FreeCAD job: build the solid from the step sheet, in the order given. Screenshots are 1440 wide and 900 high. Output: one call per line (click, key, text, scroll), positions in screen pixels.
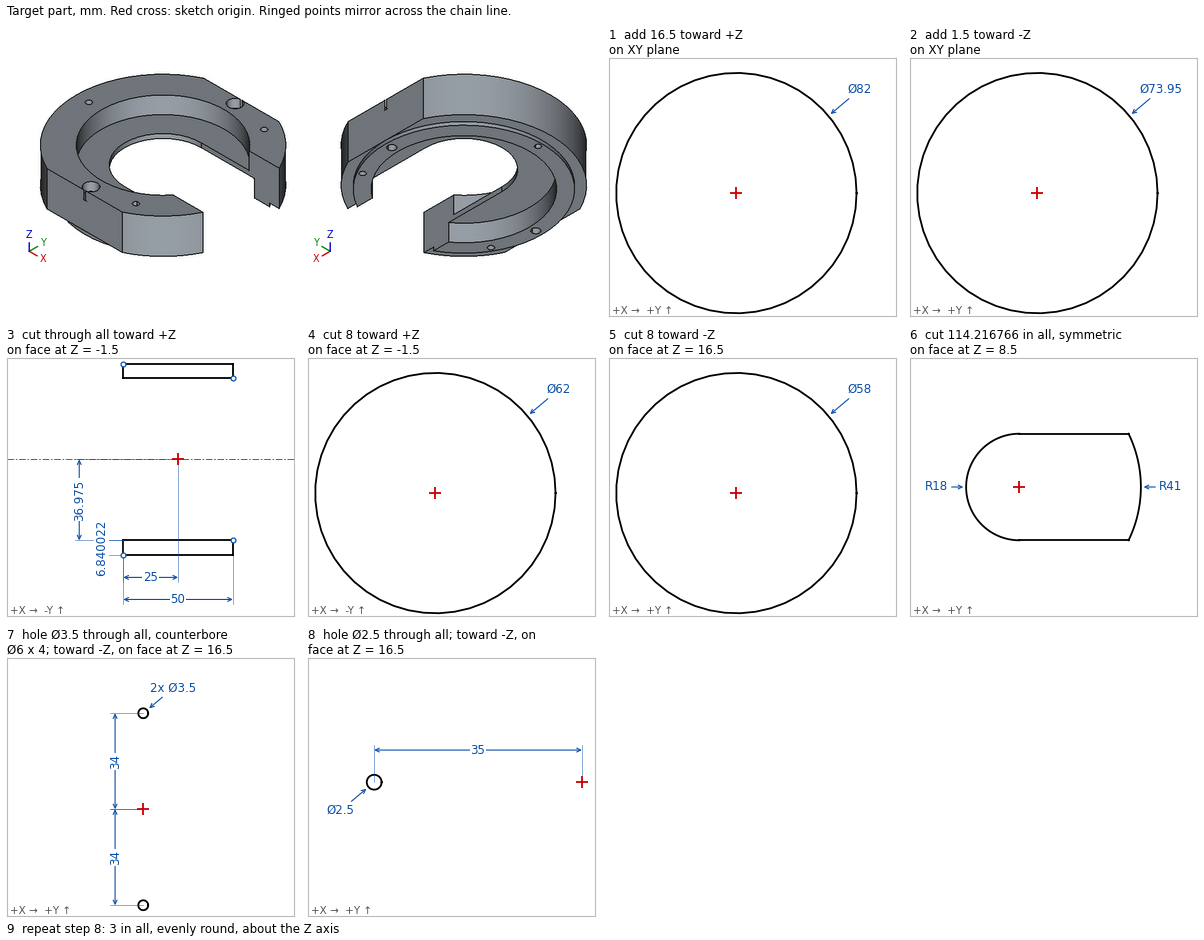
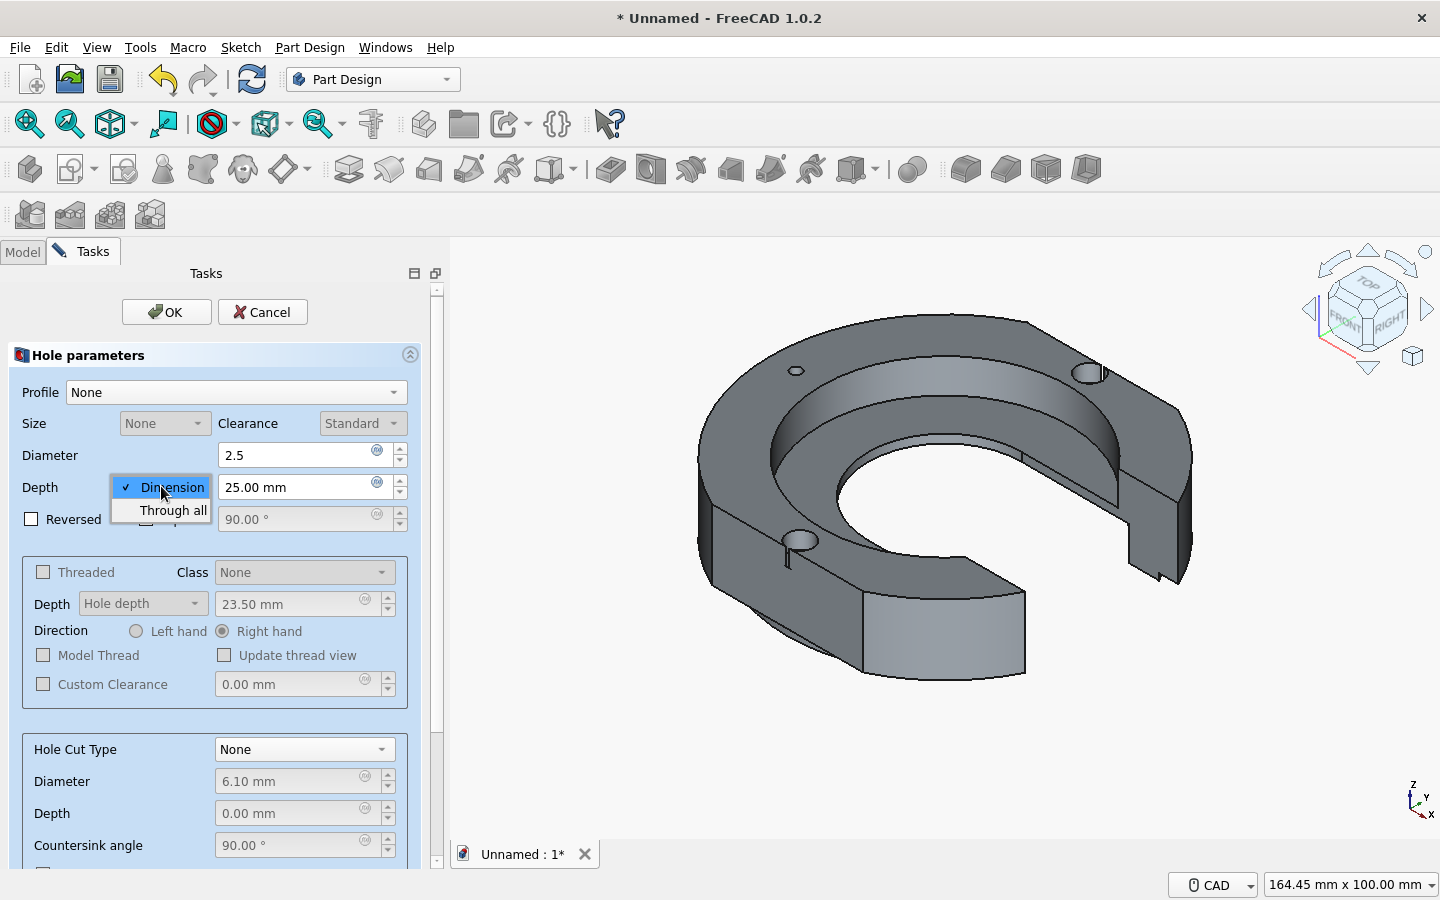
click(160, 510)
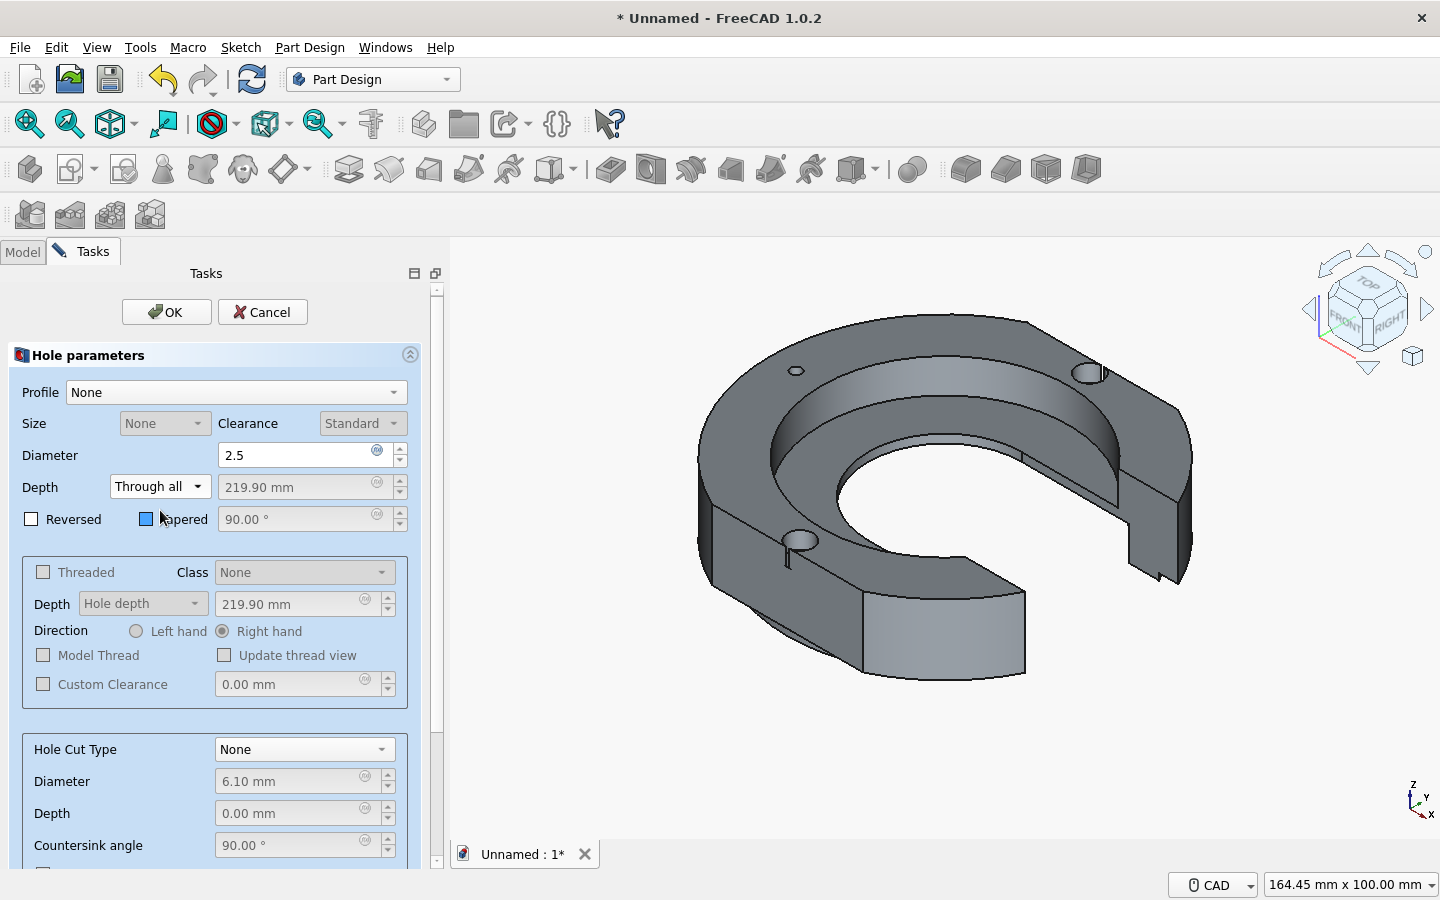
click(167, 312)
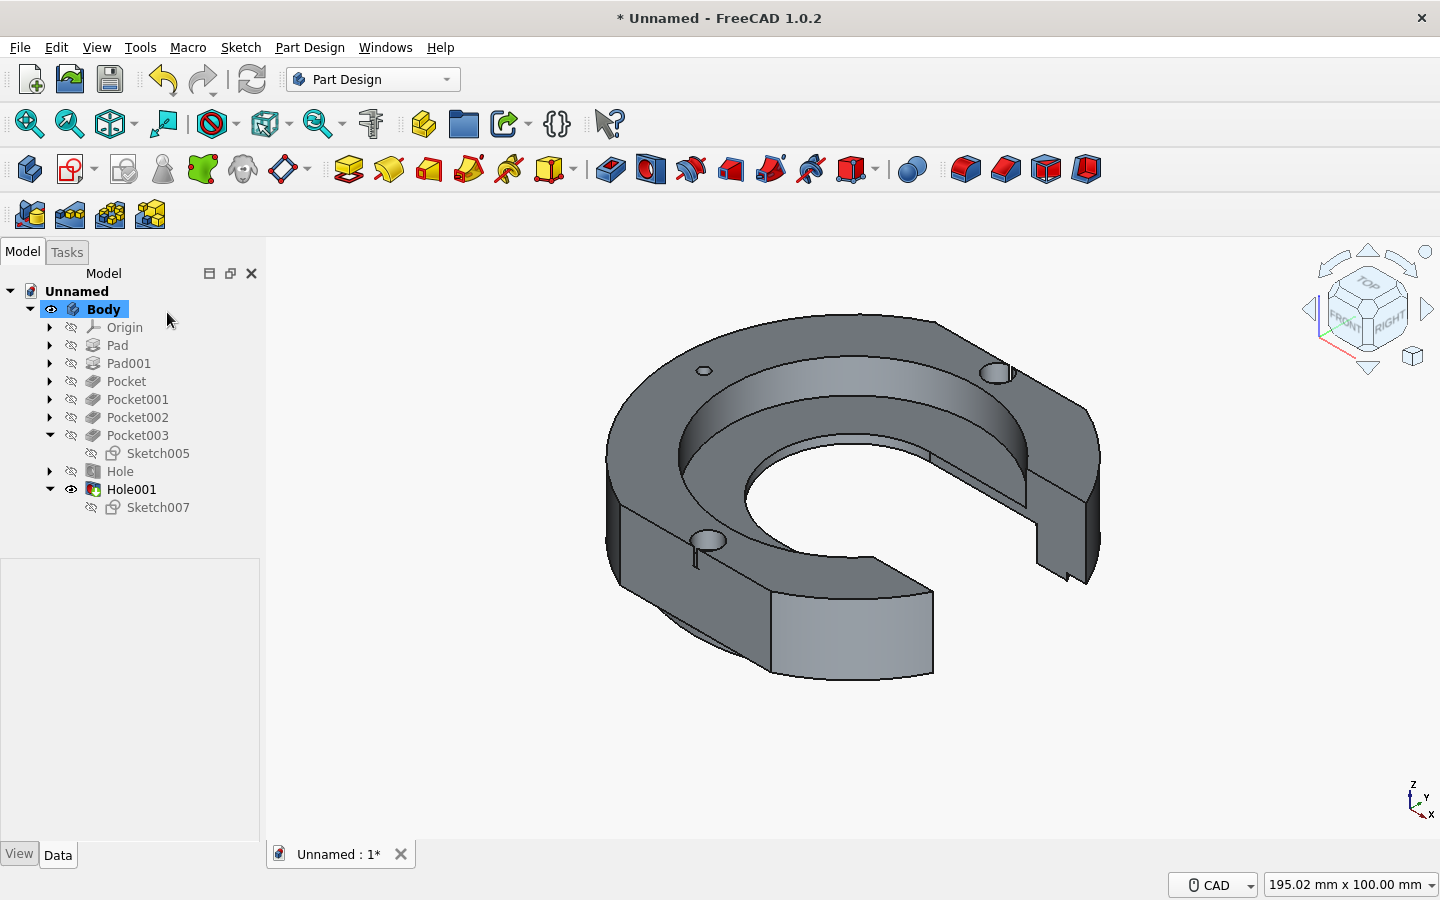
click(116, 489)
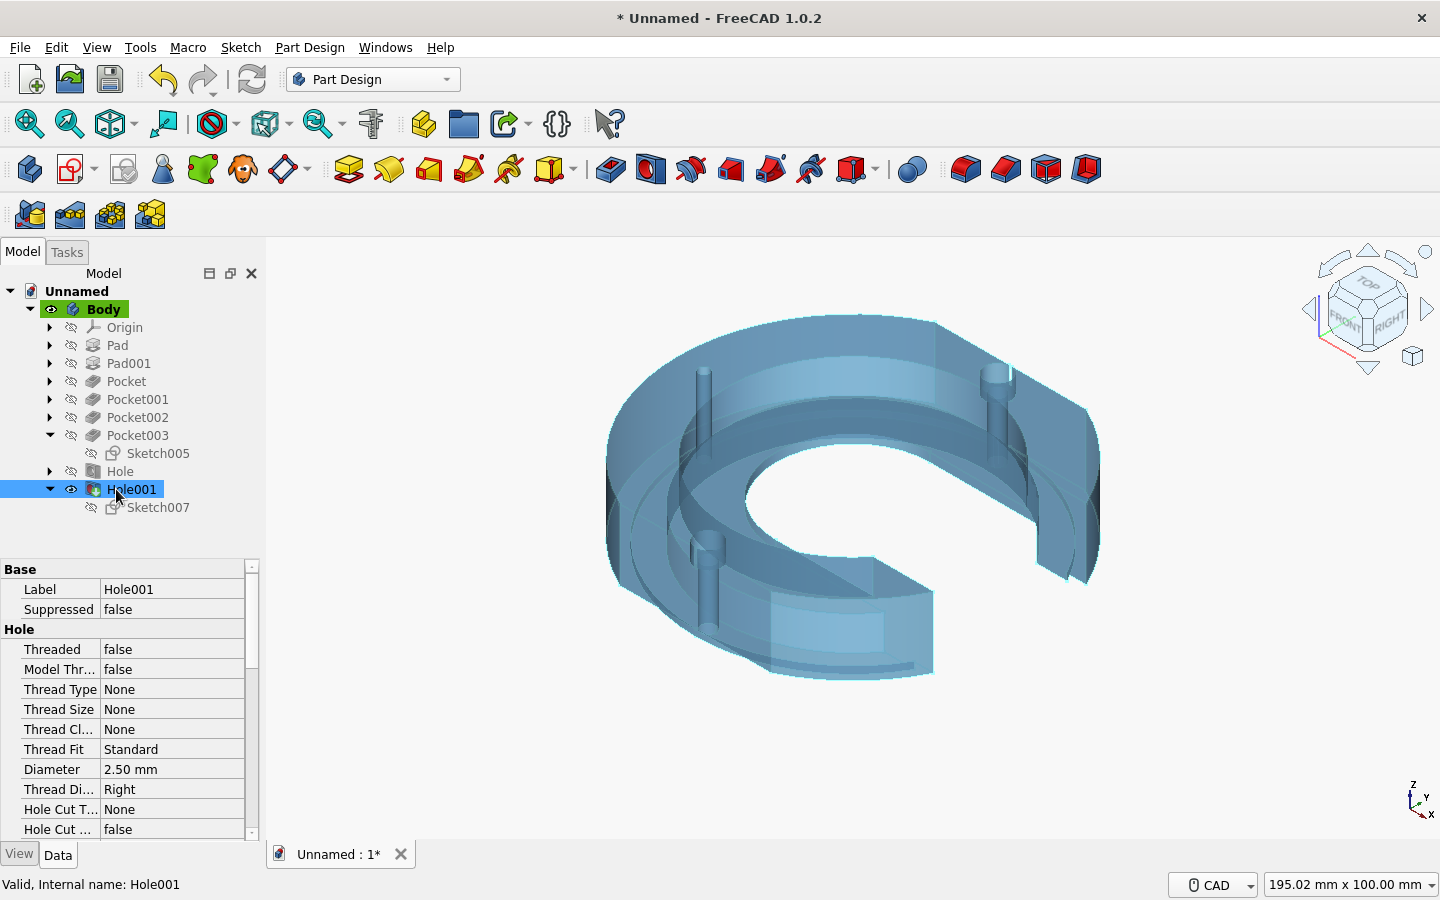
click(110, 214)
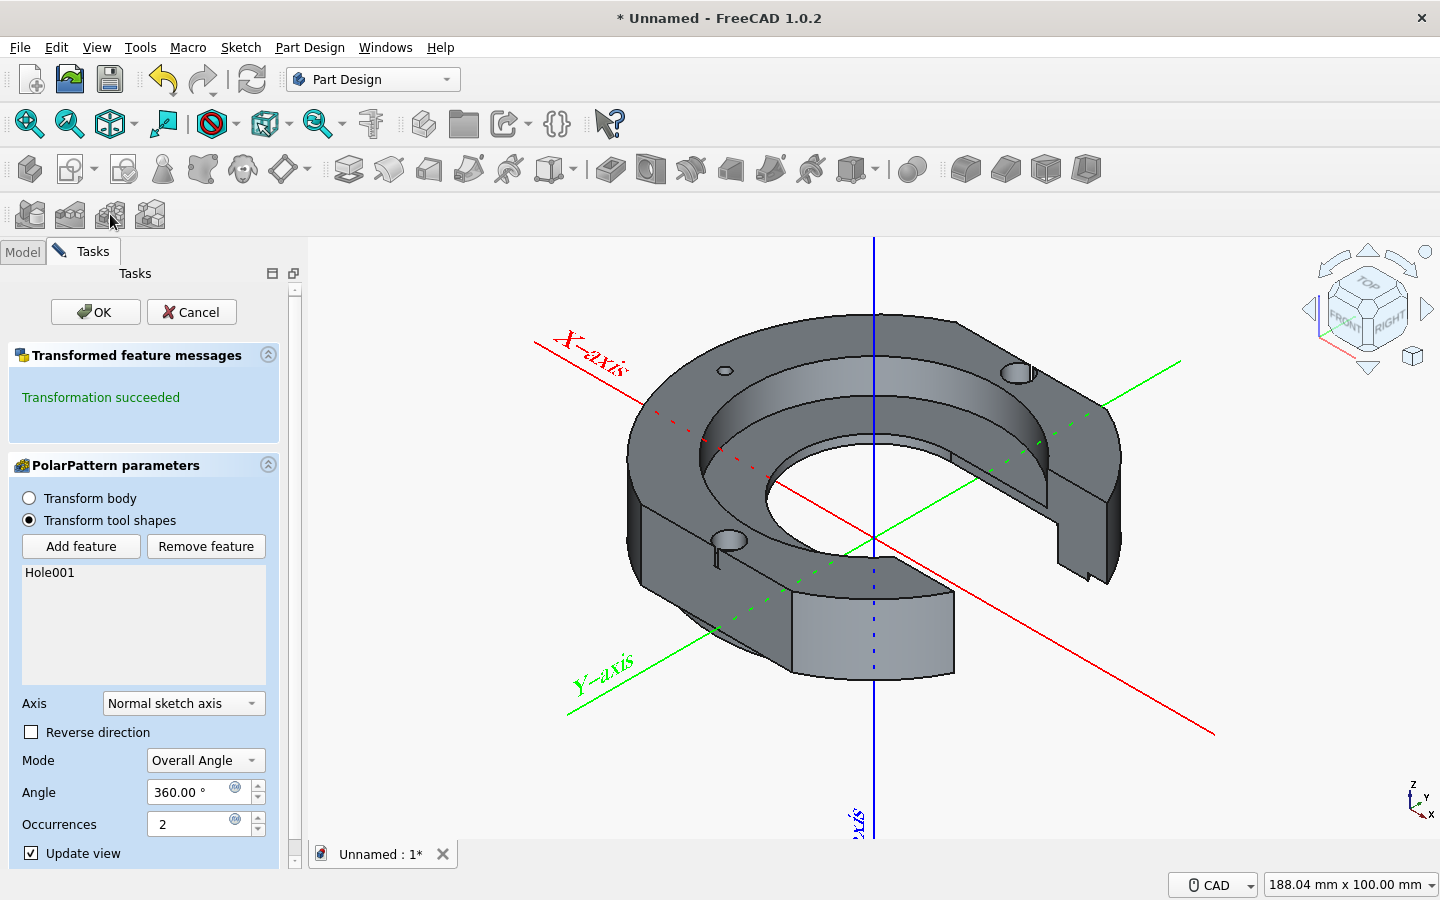
click(184, 704)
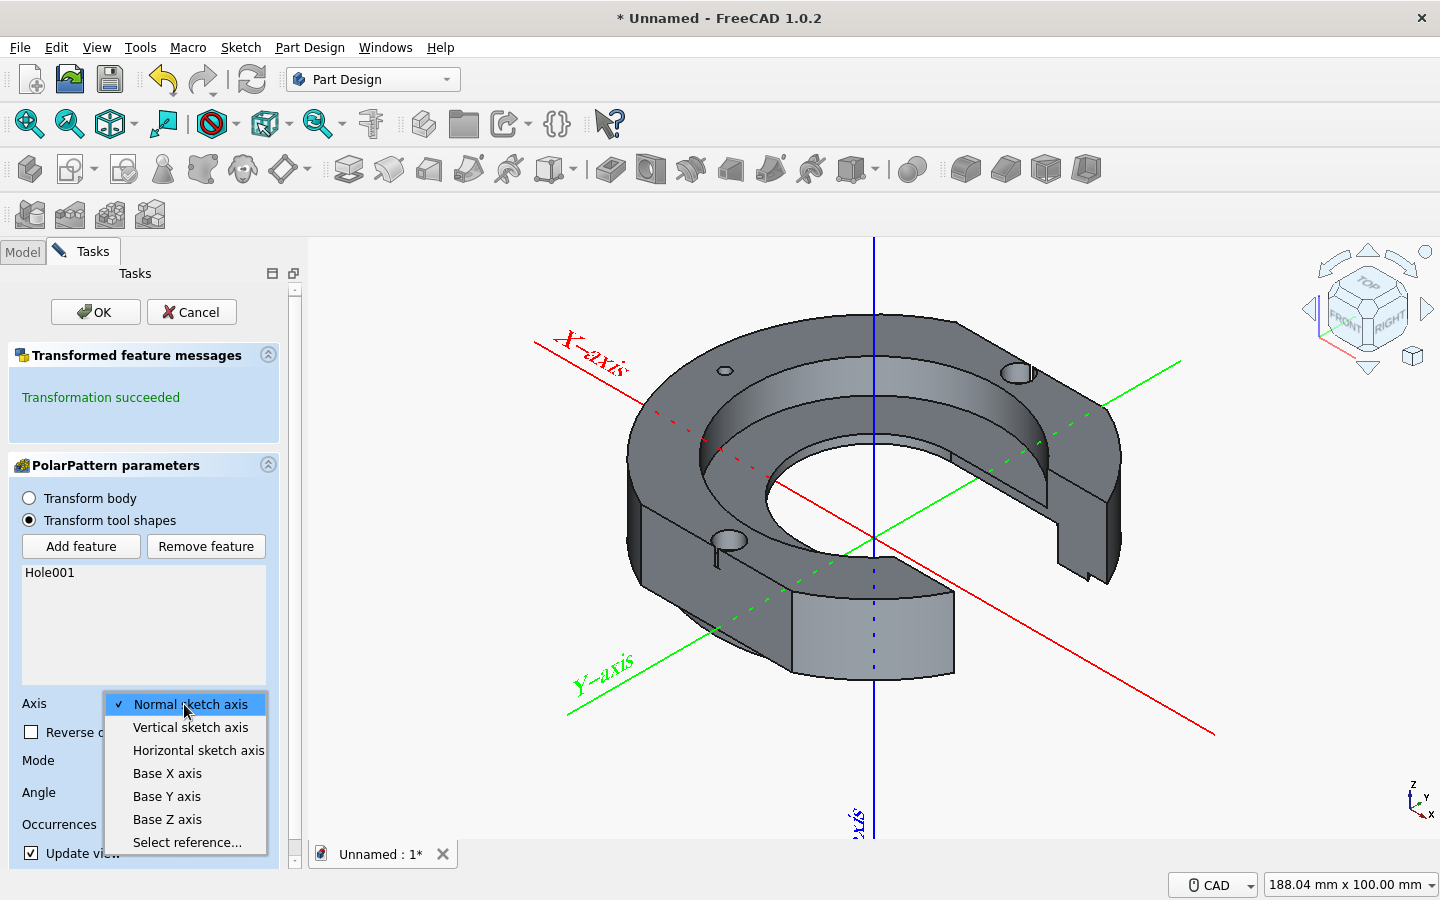
click(184, 820)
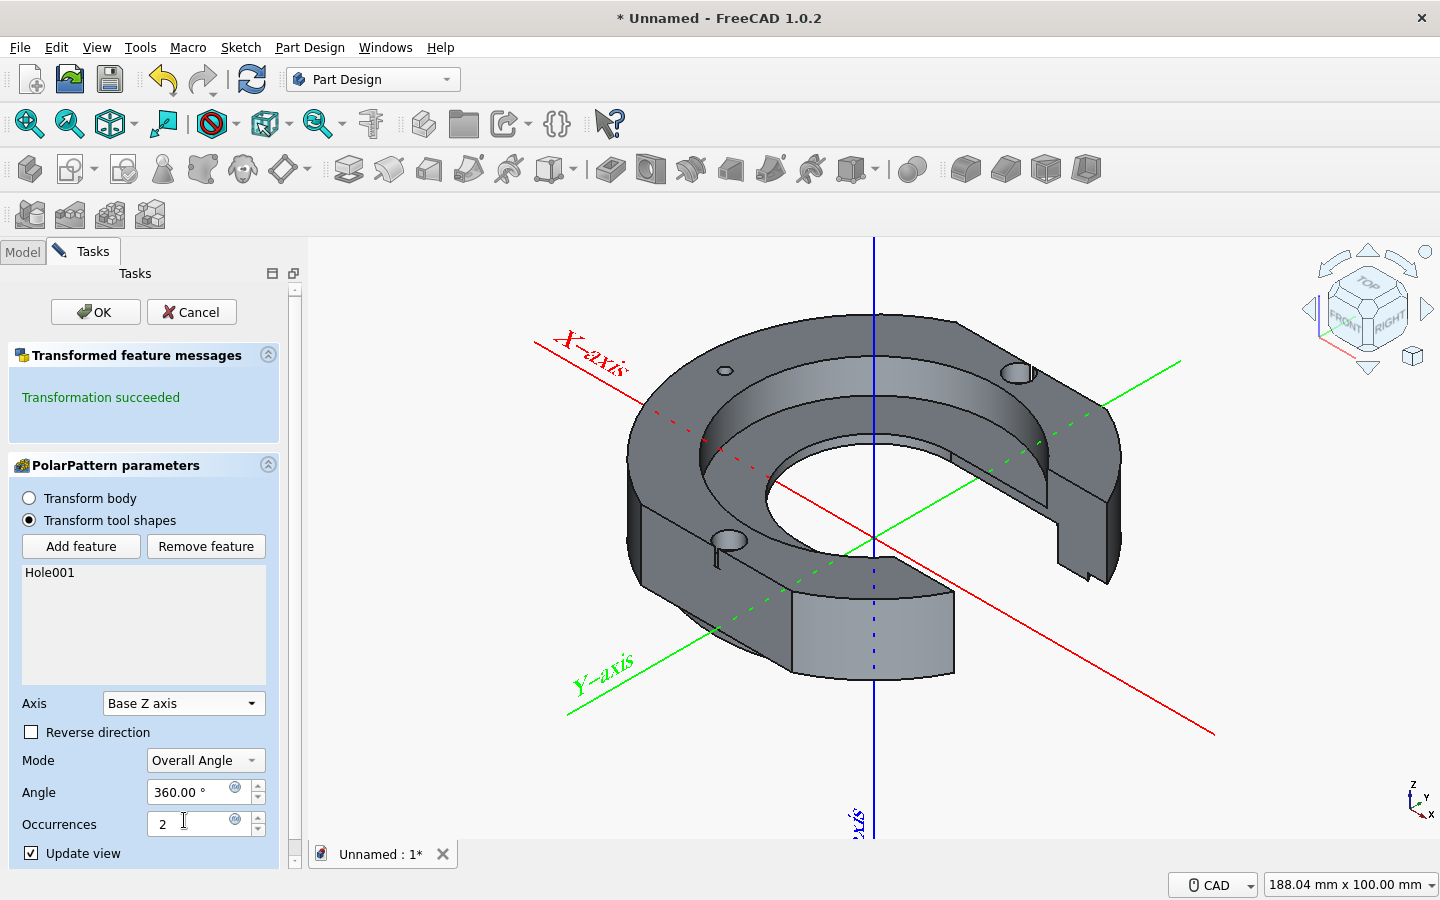
triple_click(198, 824)